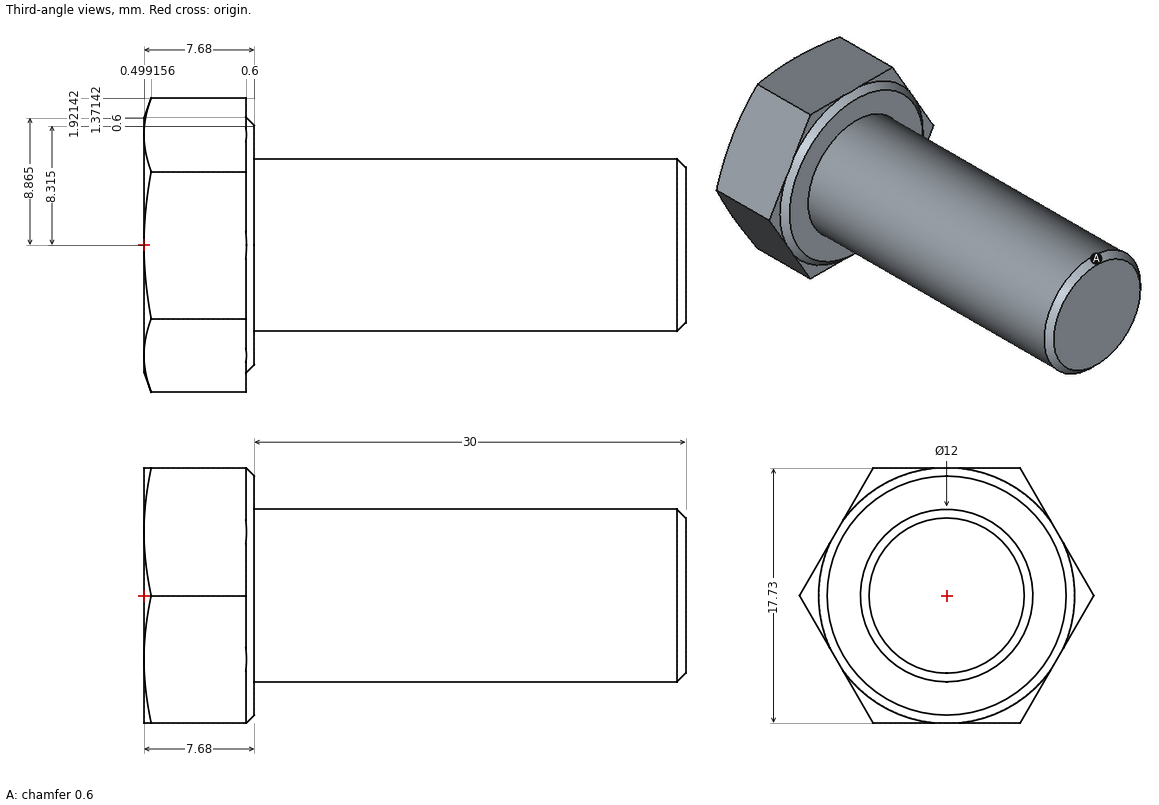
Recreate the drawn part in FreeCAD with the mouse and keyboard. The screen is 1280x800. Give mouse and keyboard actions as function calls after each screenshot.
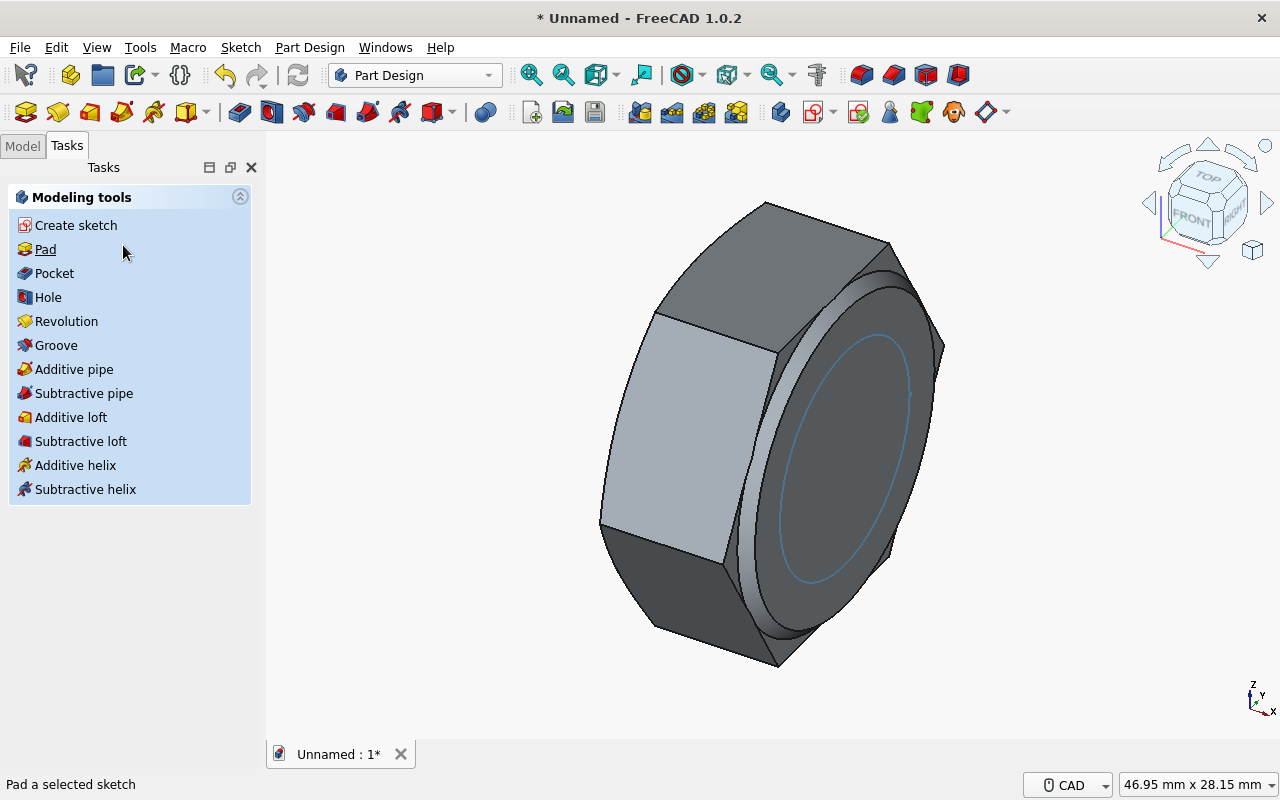
click(26, 112)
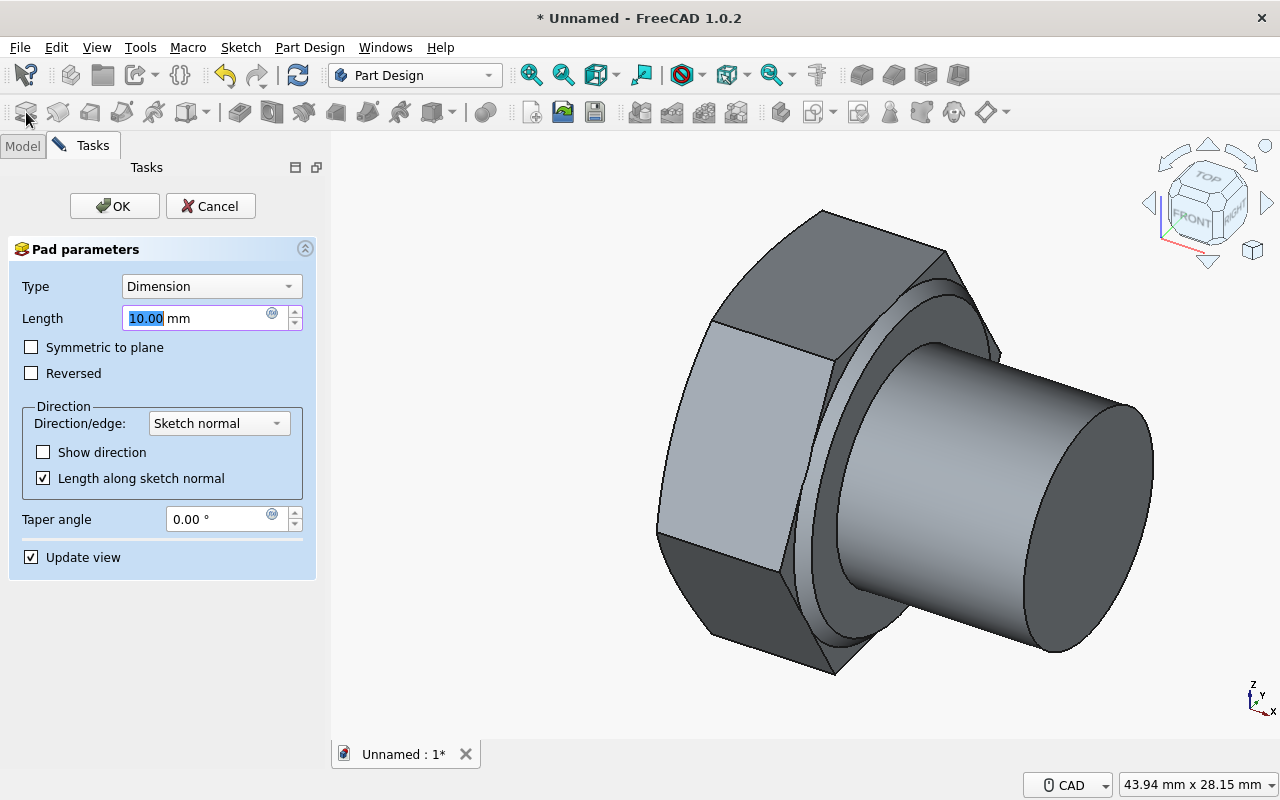
text(30)
key(Tab)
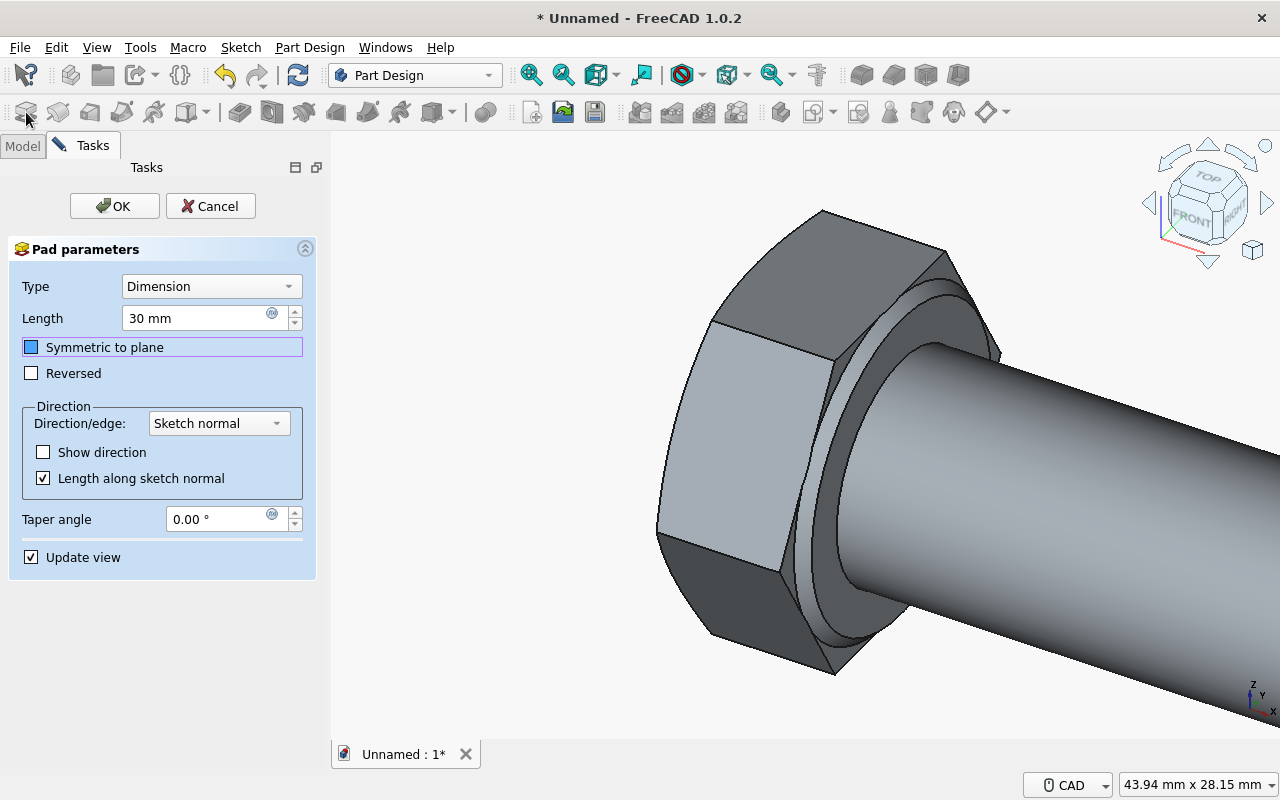
click(115, 206)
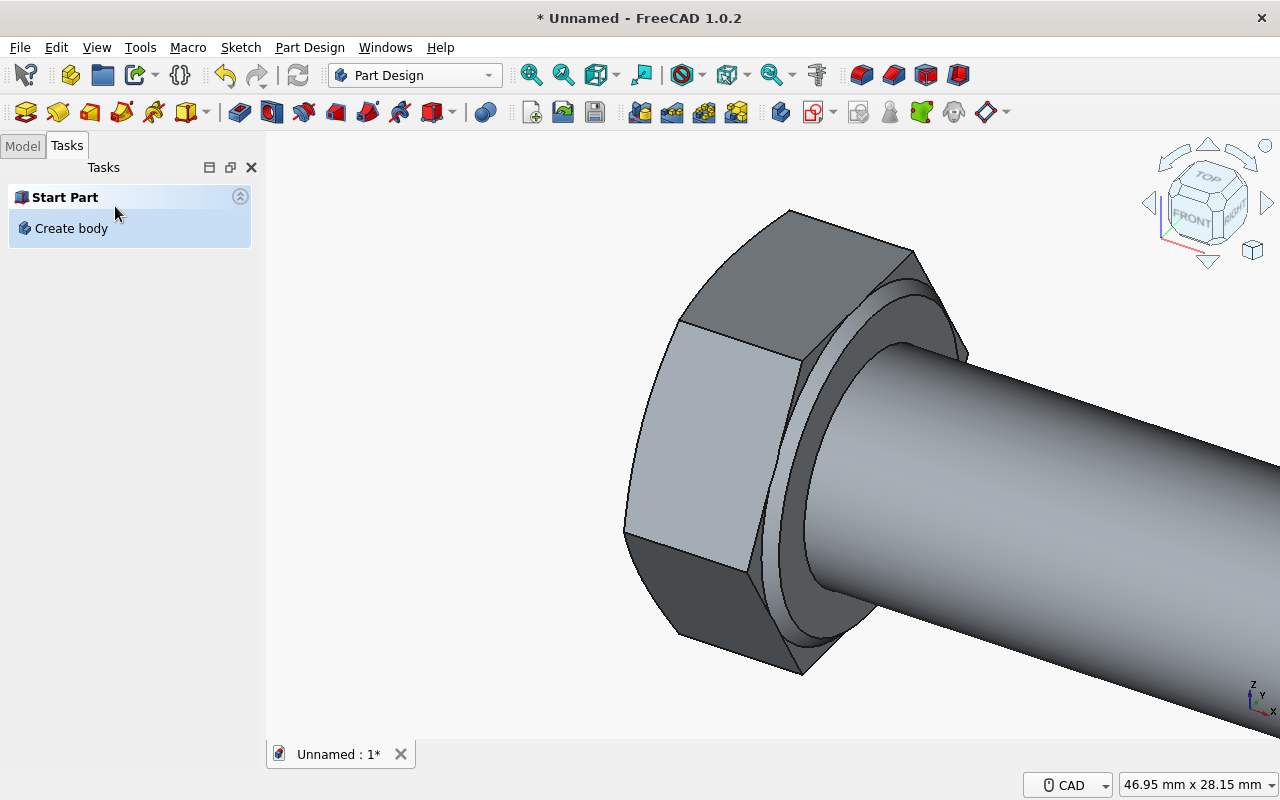
click(532, 76)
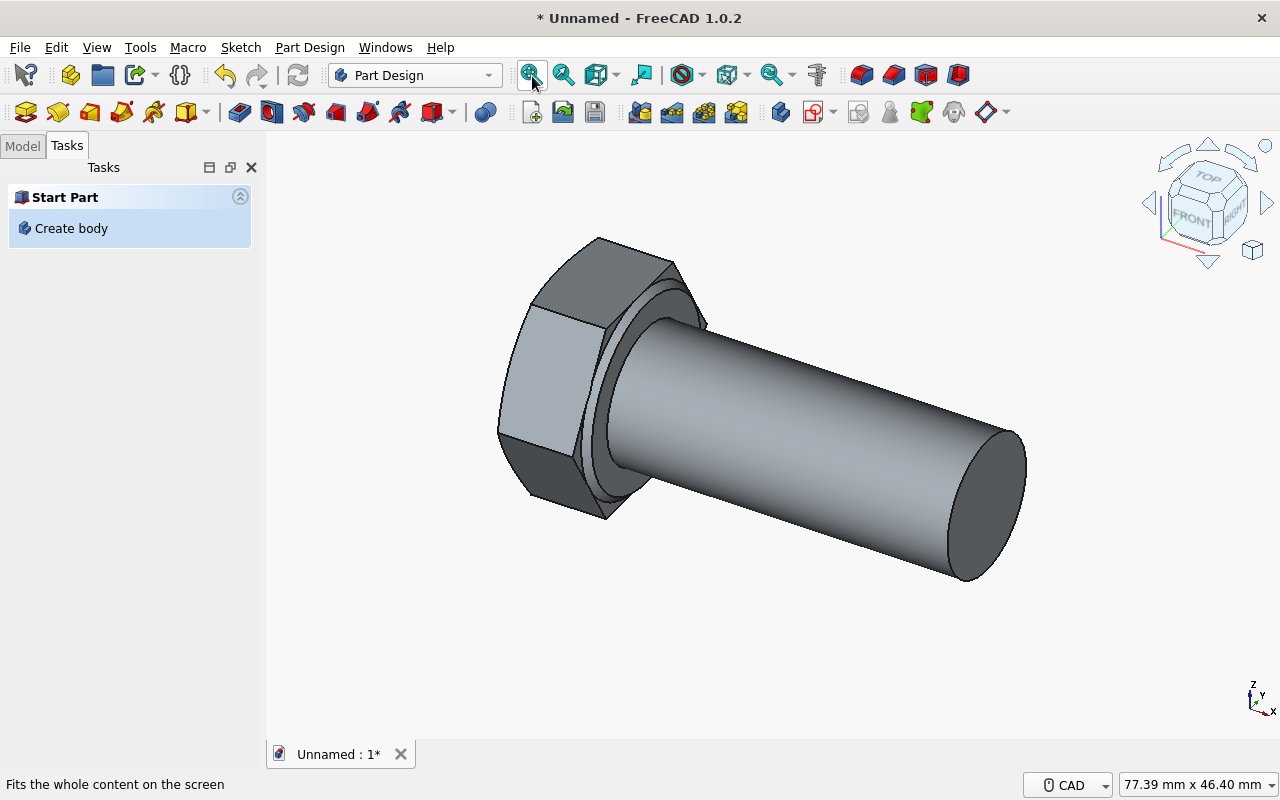
click(947, 544)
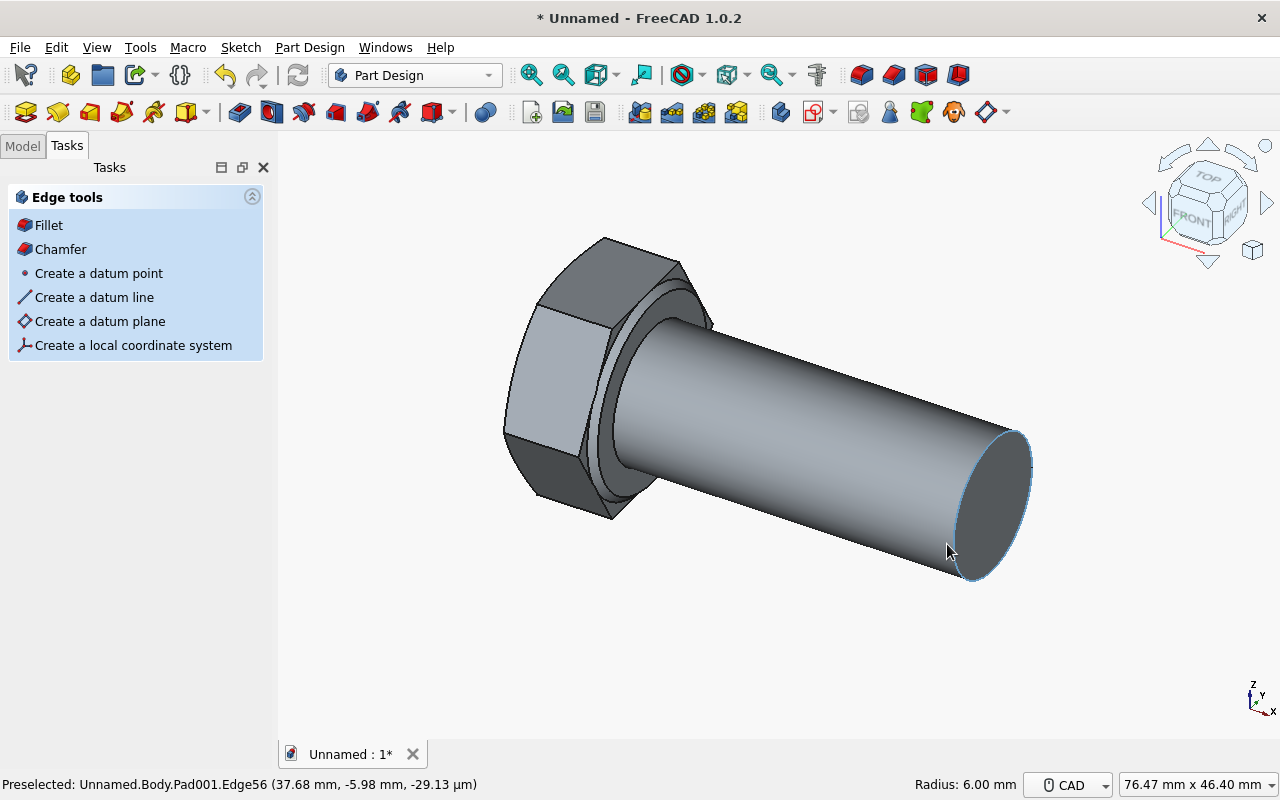
click(894, 76)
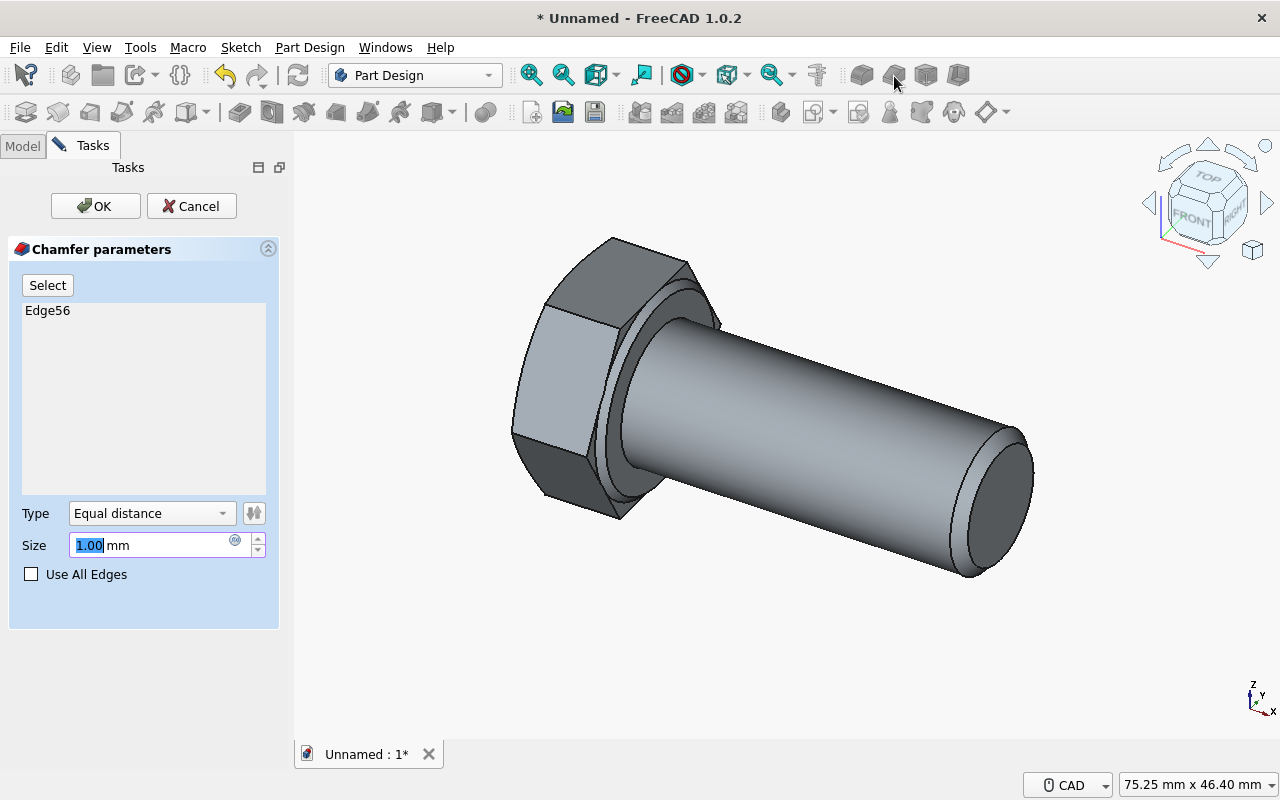
text(0.6)
key(Tab)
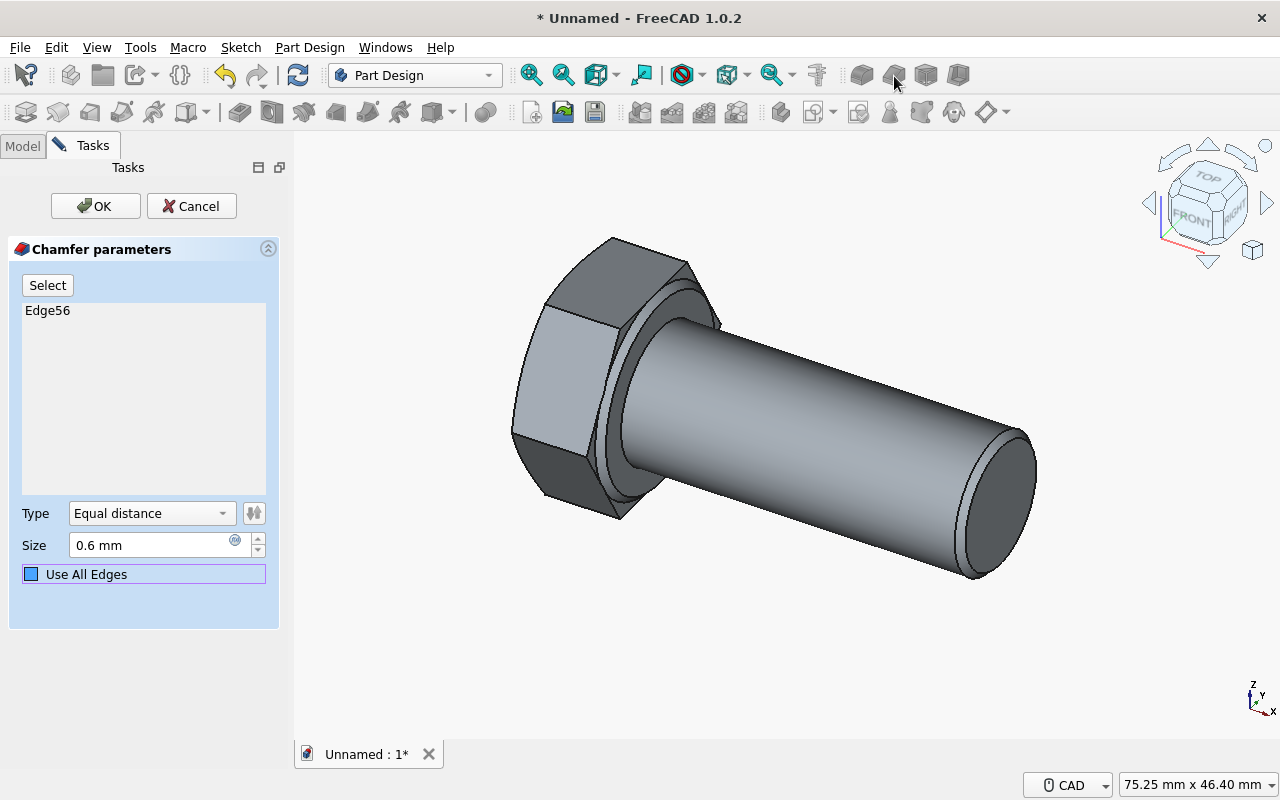
click(96, 206)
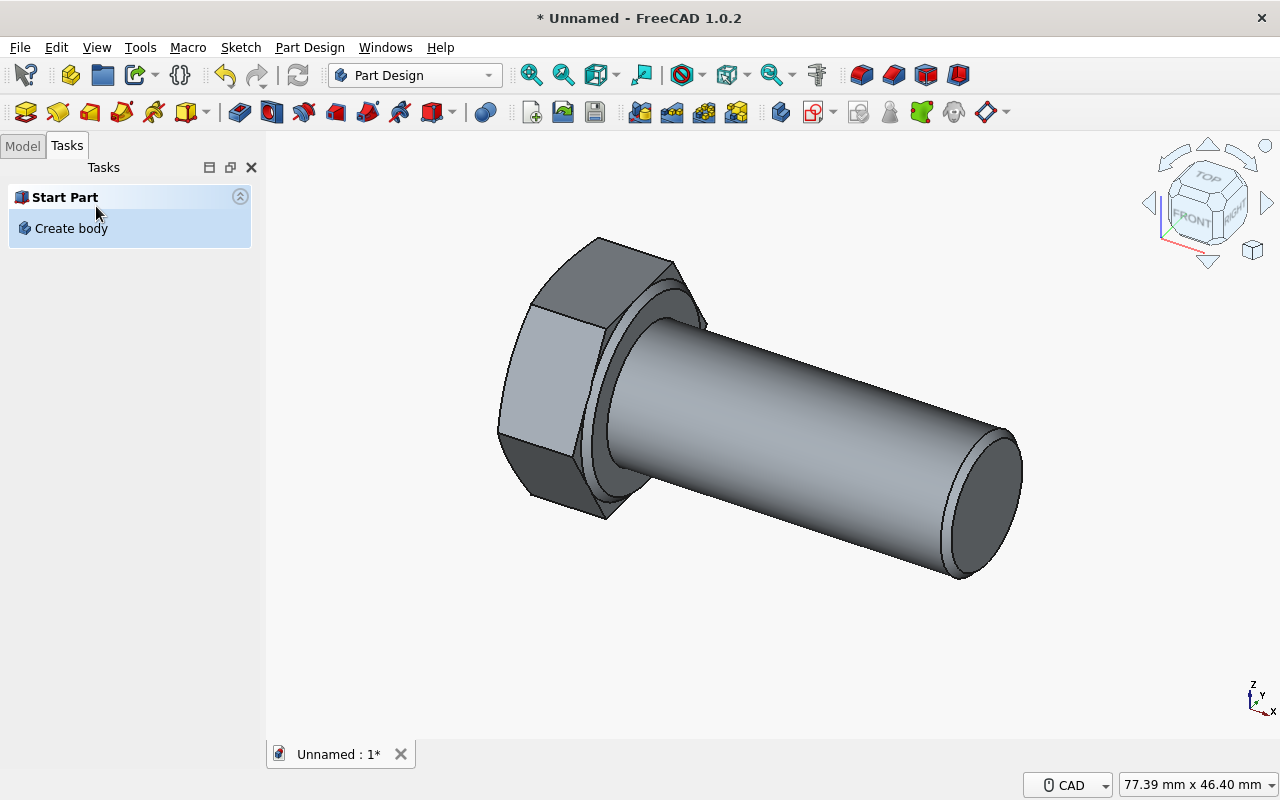
key(0)